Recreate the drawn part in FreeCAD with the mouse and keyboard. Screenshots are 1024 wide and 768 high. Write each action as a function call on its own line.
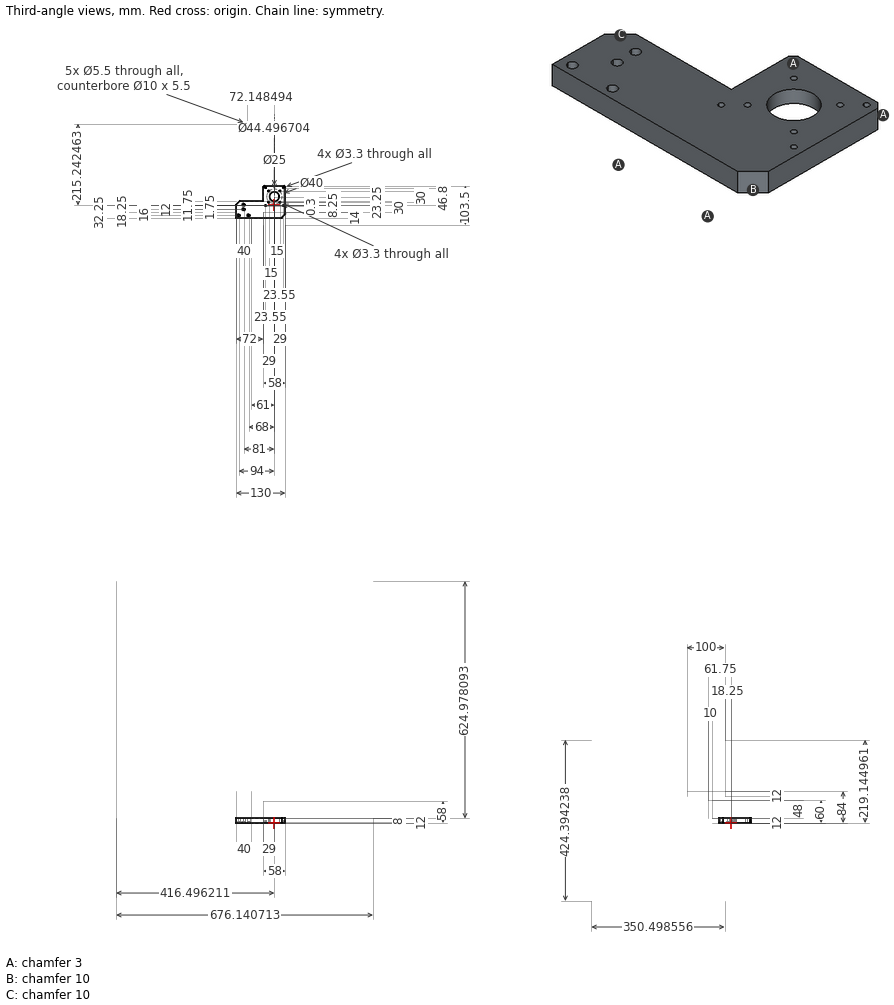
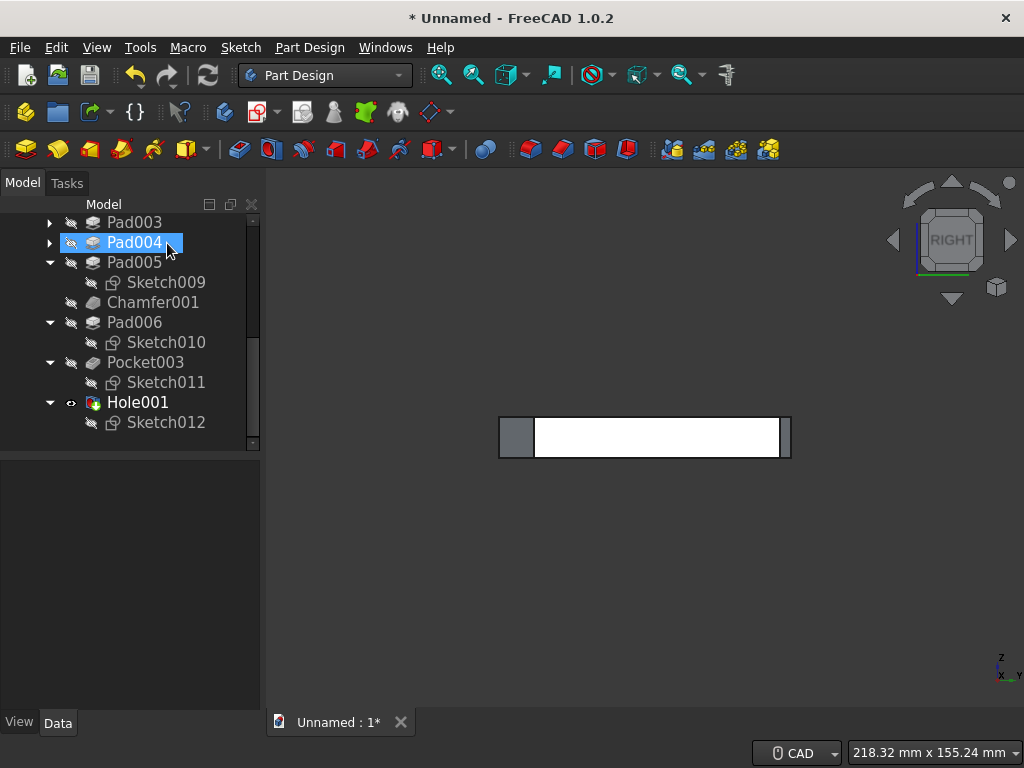
key(5)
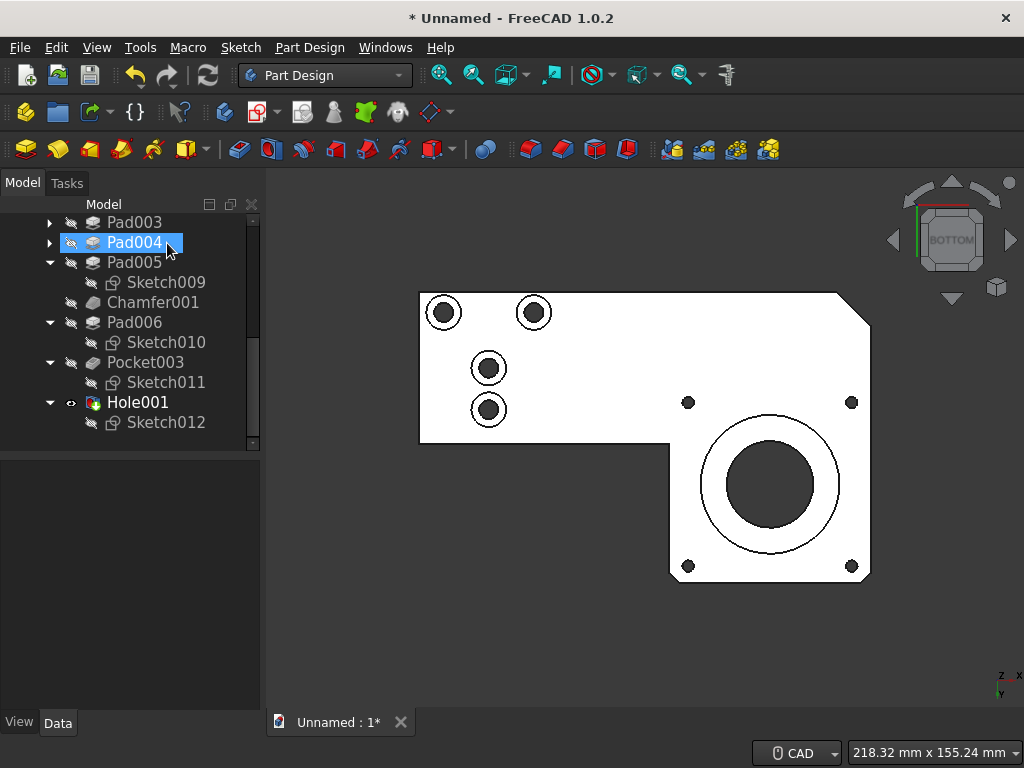
key(4)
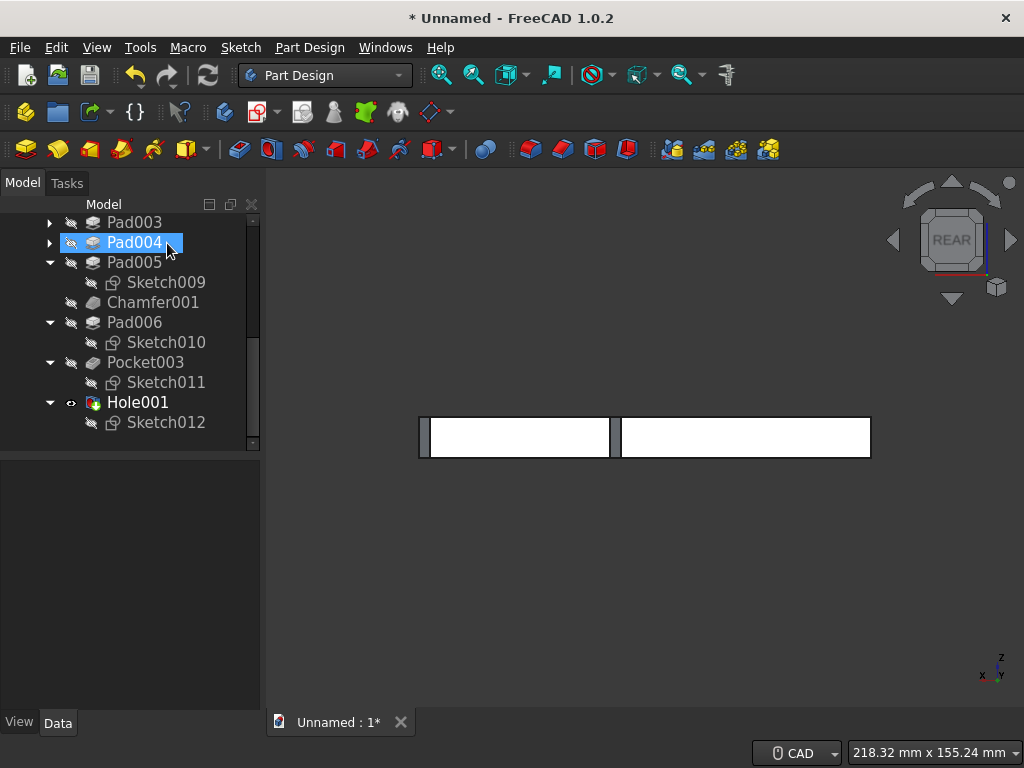
click(871, 436)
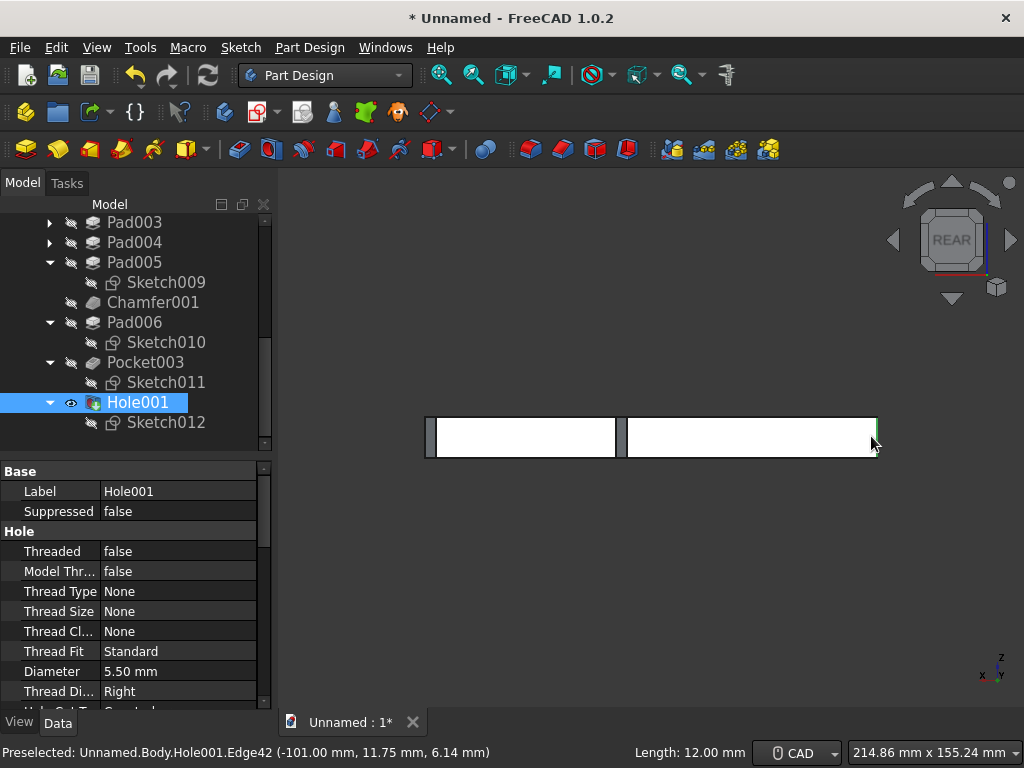
click(564, 150)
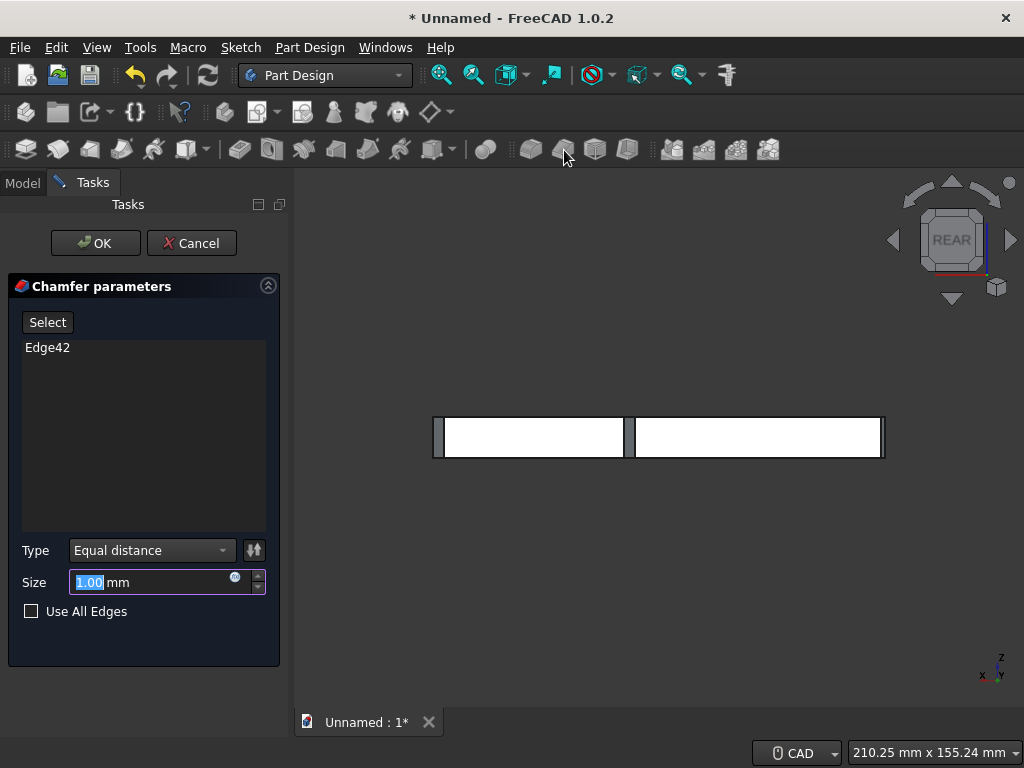
text(10)
key(Tab)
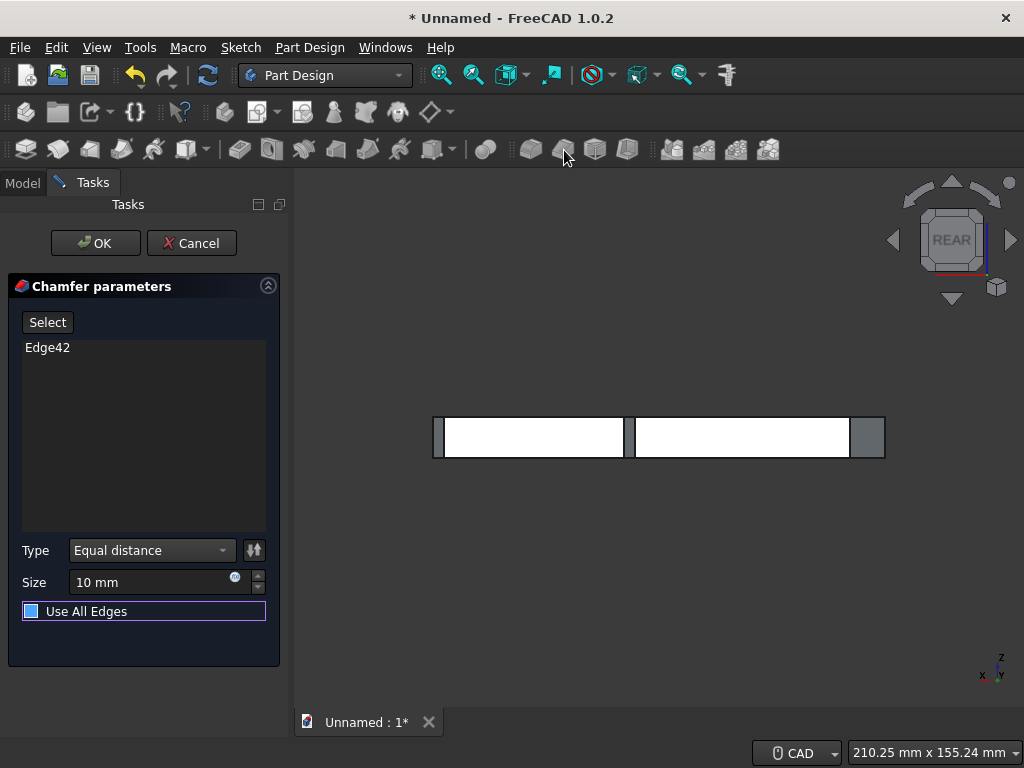
click(96, 243)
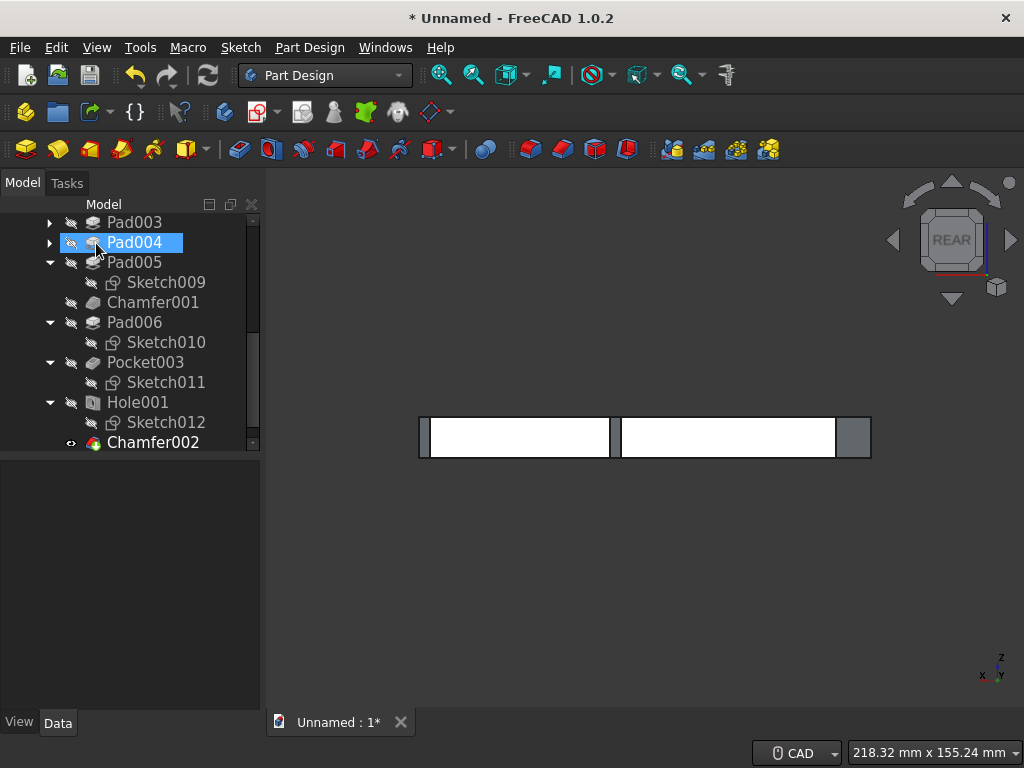
key(0)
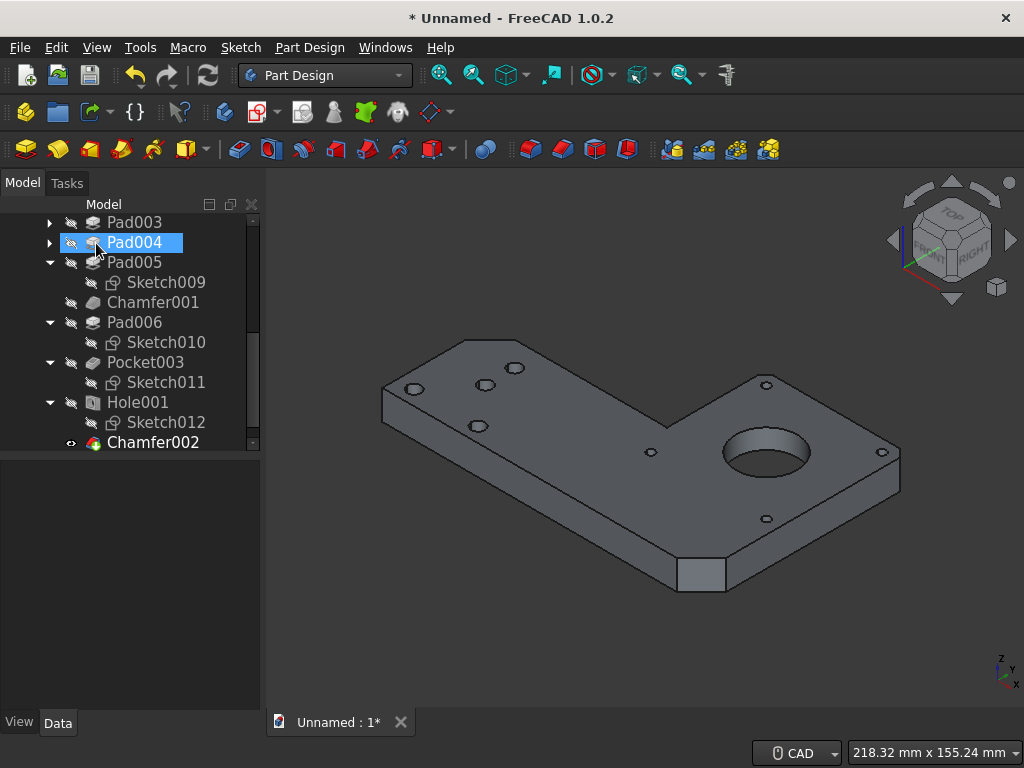
click(677, 506)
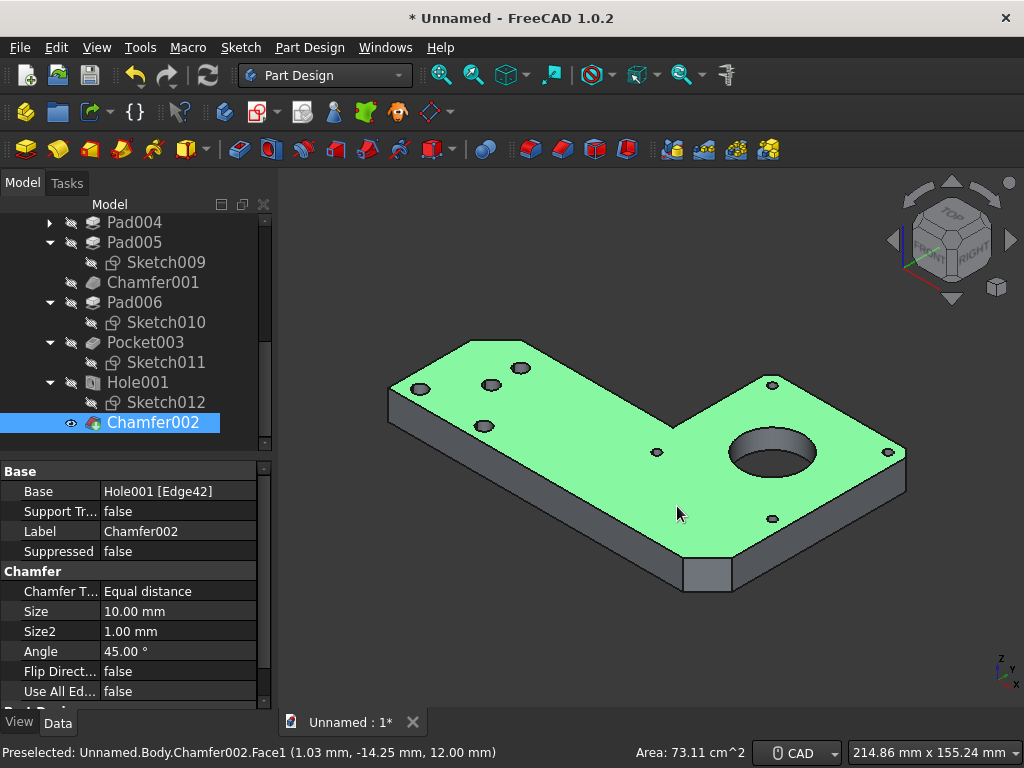
click(258, 112)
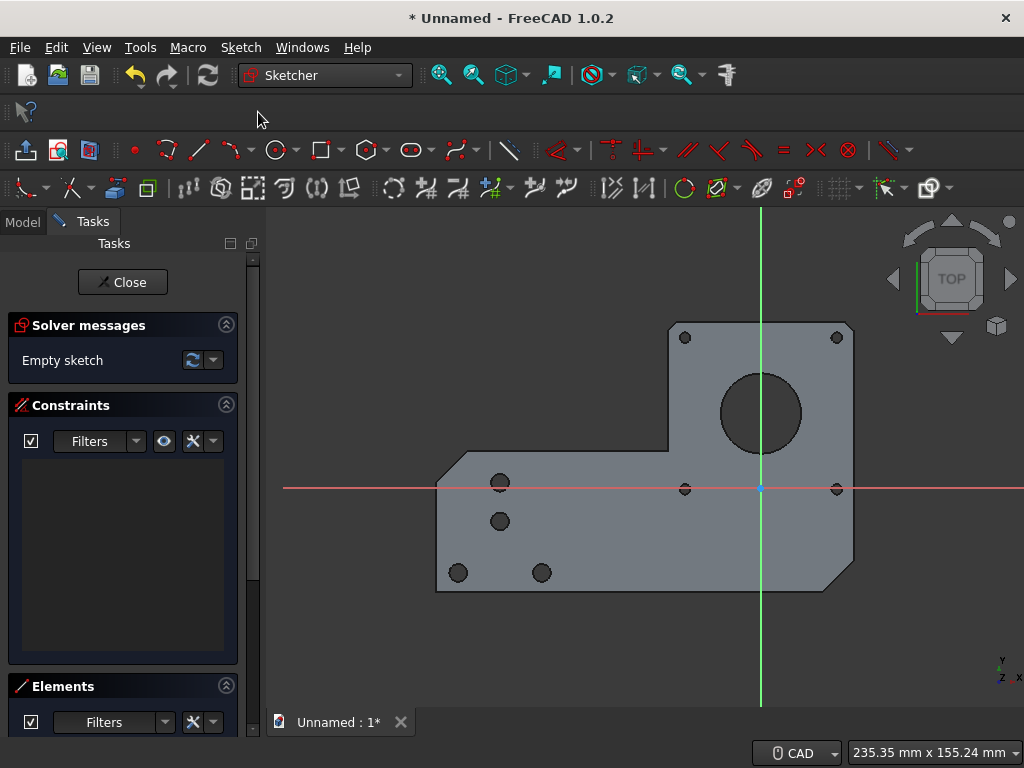
scroll(859, 397, up, 4)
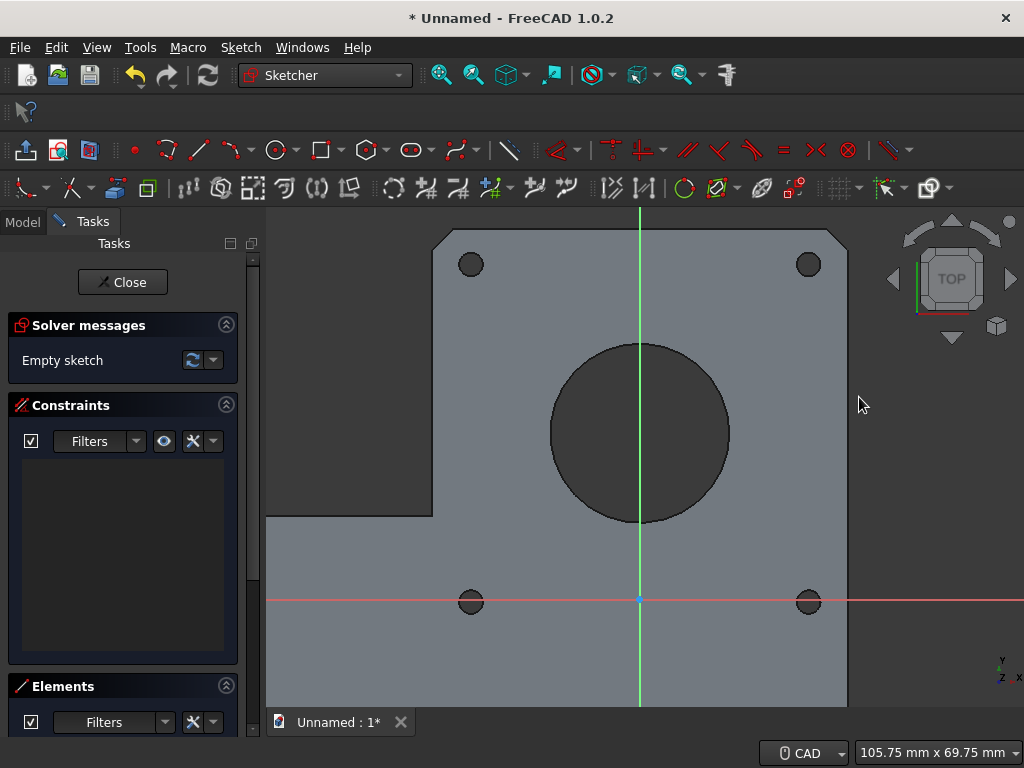
key(g)
key(c)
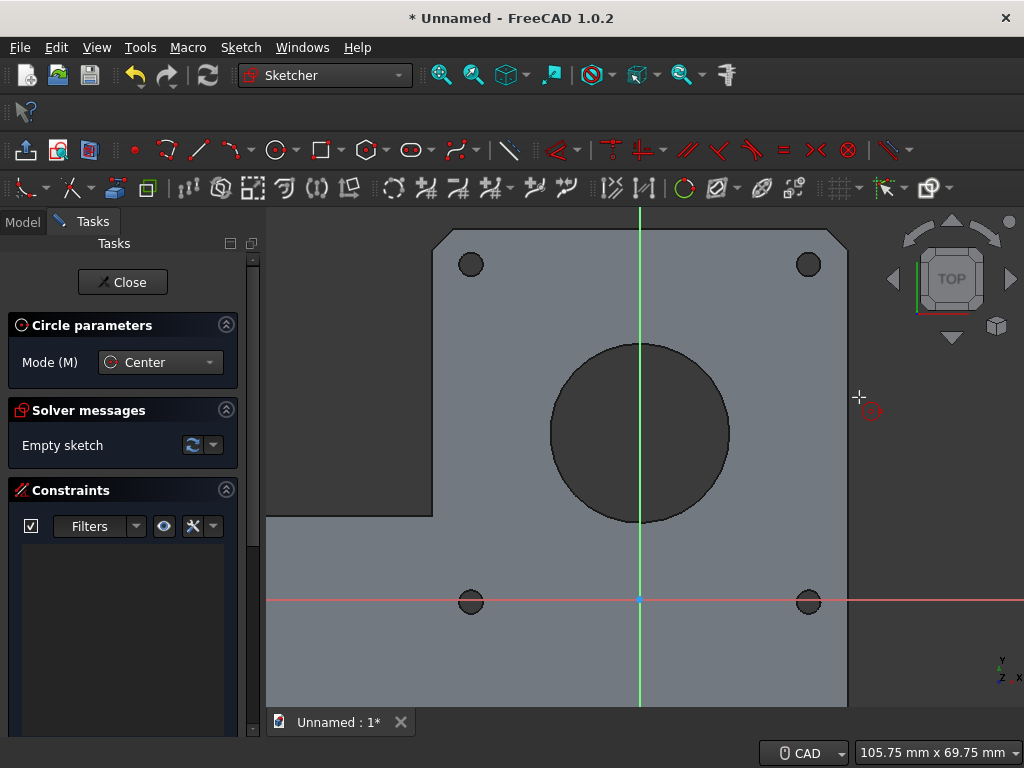
scroll(747, 541, up, 4)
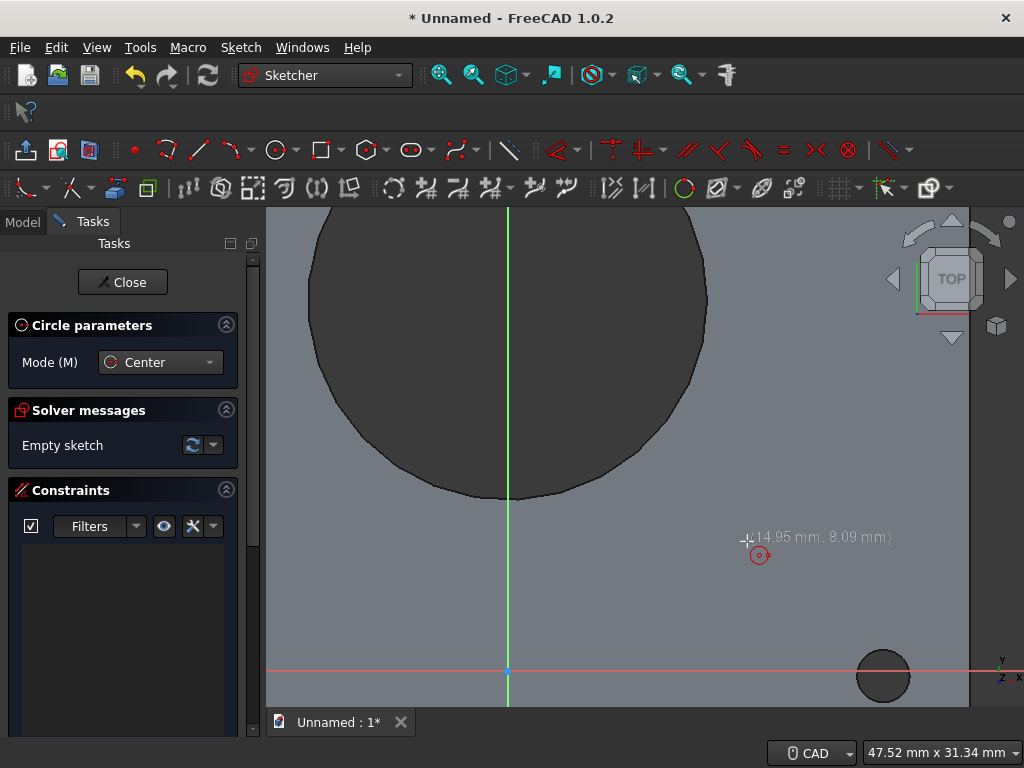
click(747, 540)
move(766, 521)